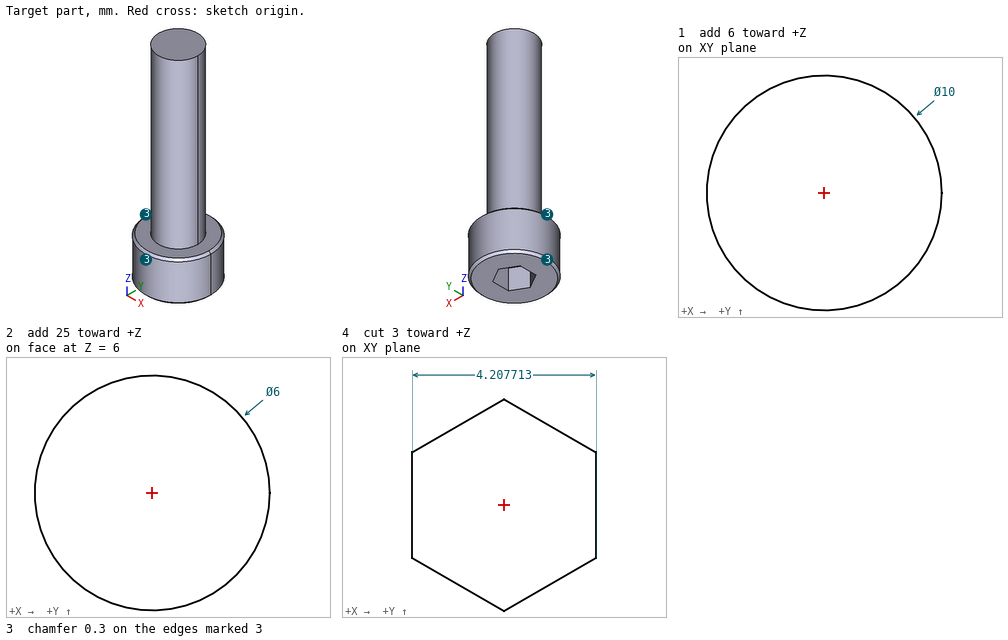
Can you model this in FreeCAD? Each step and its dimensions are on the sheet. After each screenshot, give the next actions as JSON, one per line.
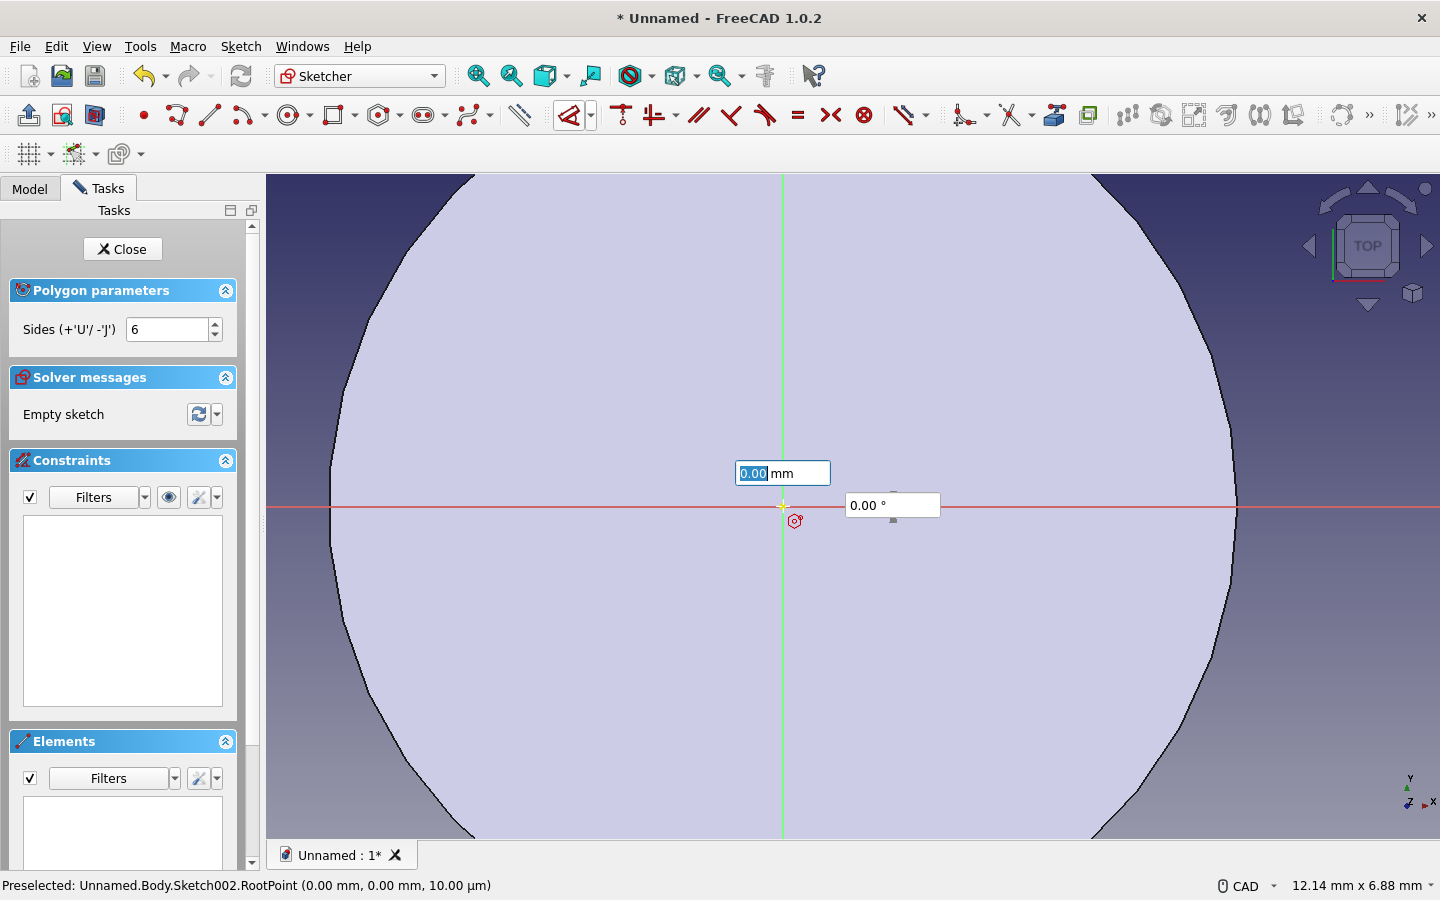
{"action": "left_click", "coordinate": [783, 272]}
{"action": "right_click", "coordinate": [783, 272]}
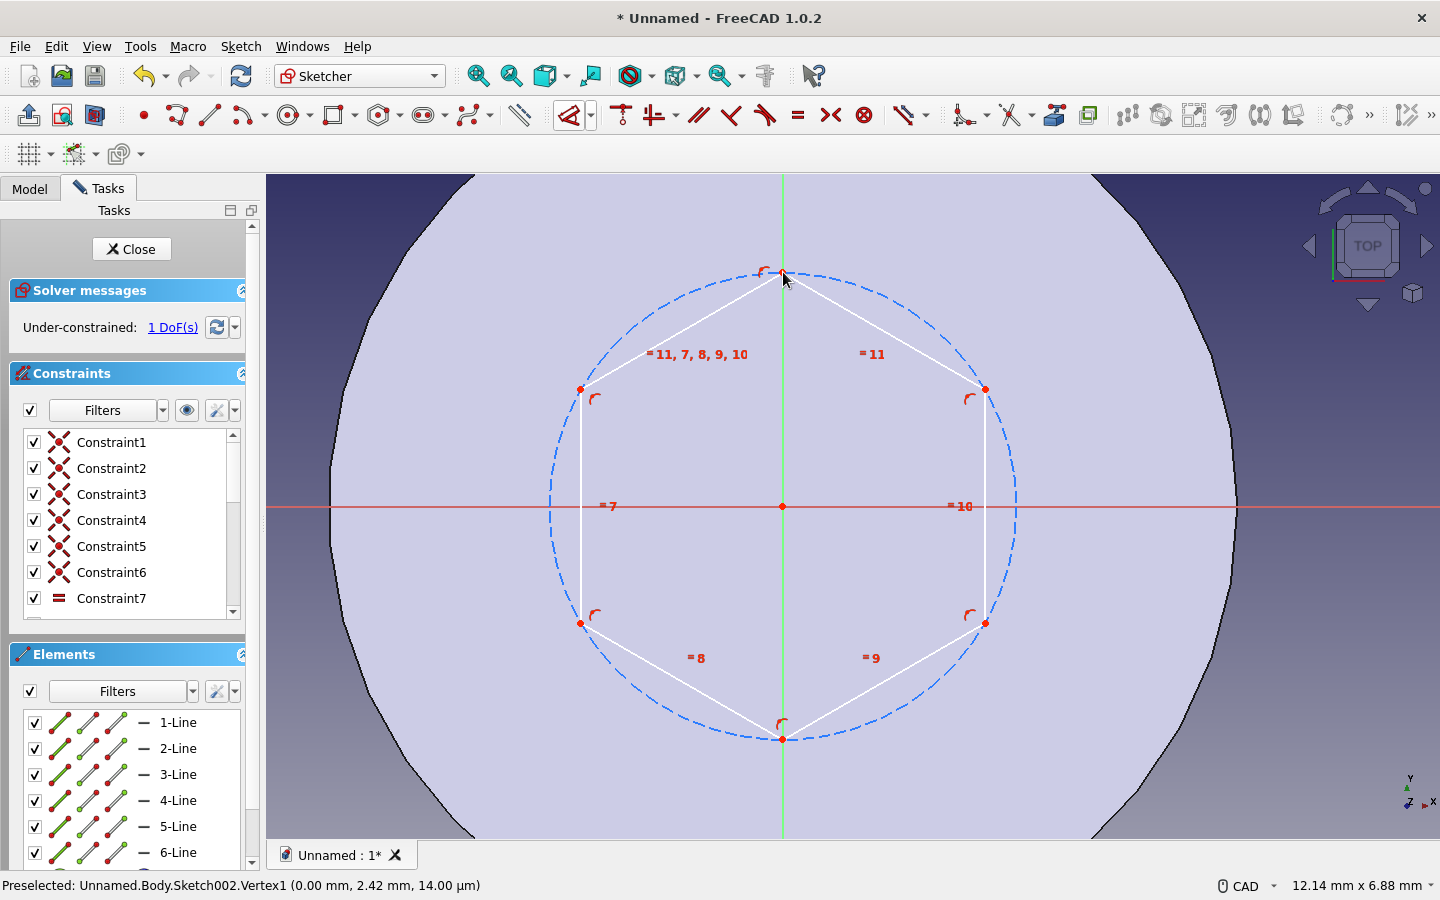
{"action": "key", "text": "d"}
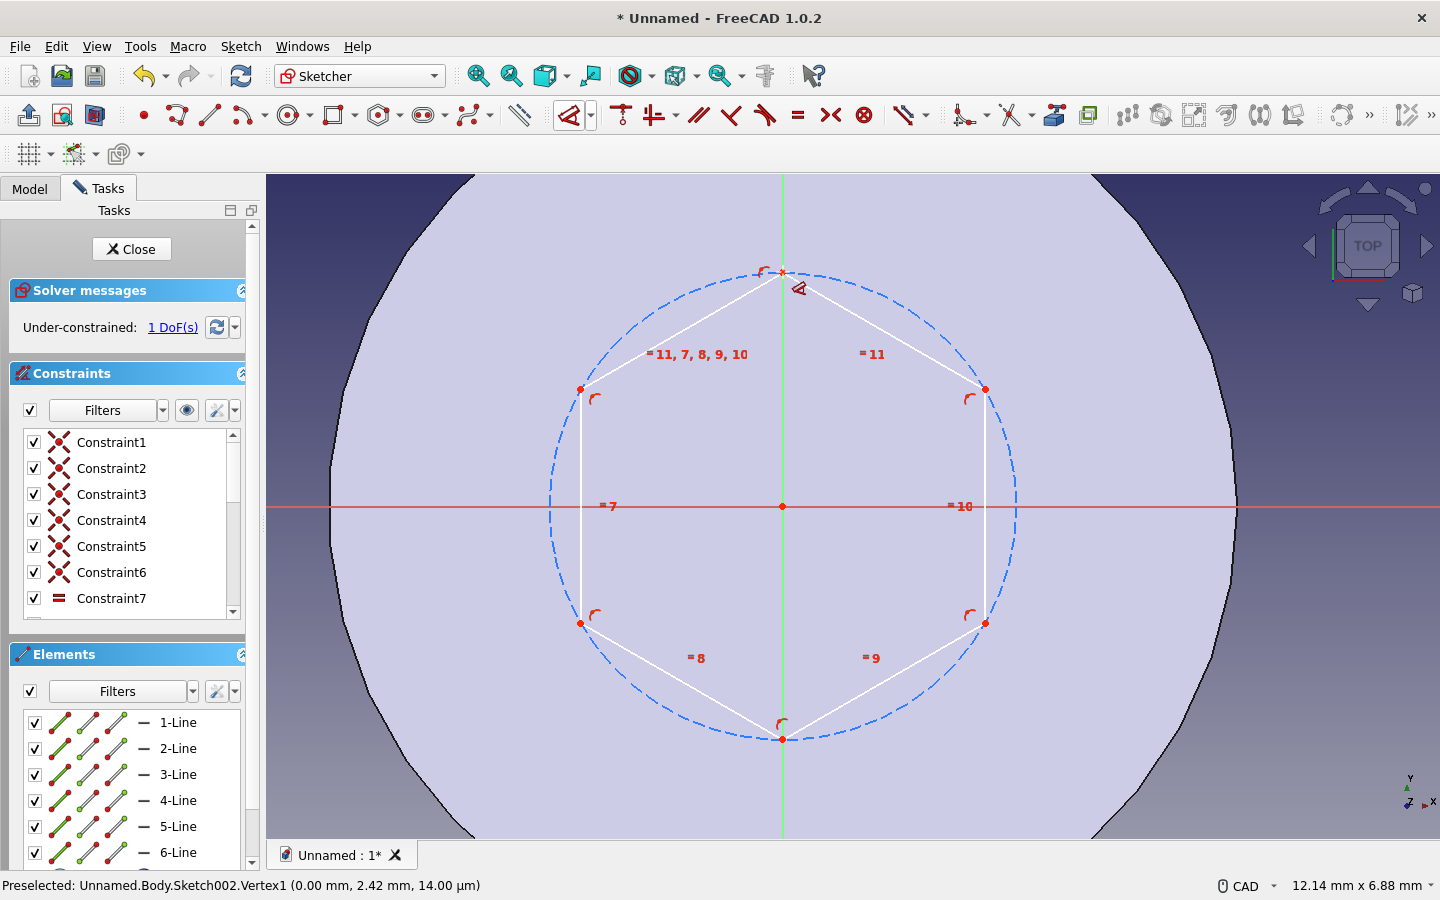
{"action": "left_click", "coordinate": [581, 390]}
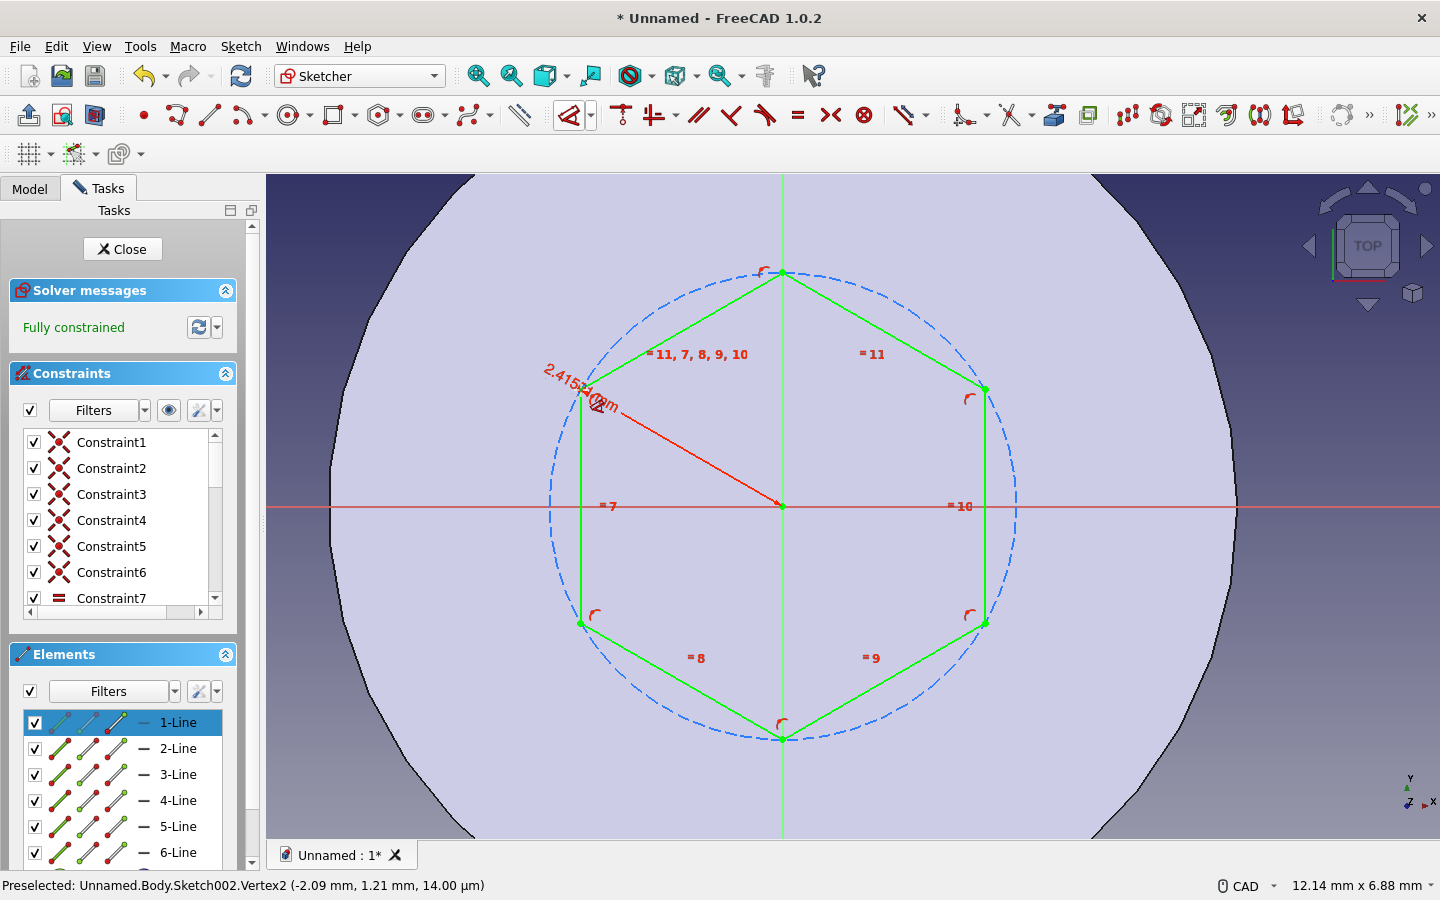
{"action": "left_click", "coordinate": [985, 623]}
{"action": "left_click", "coordinate": [690, 657]}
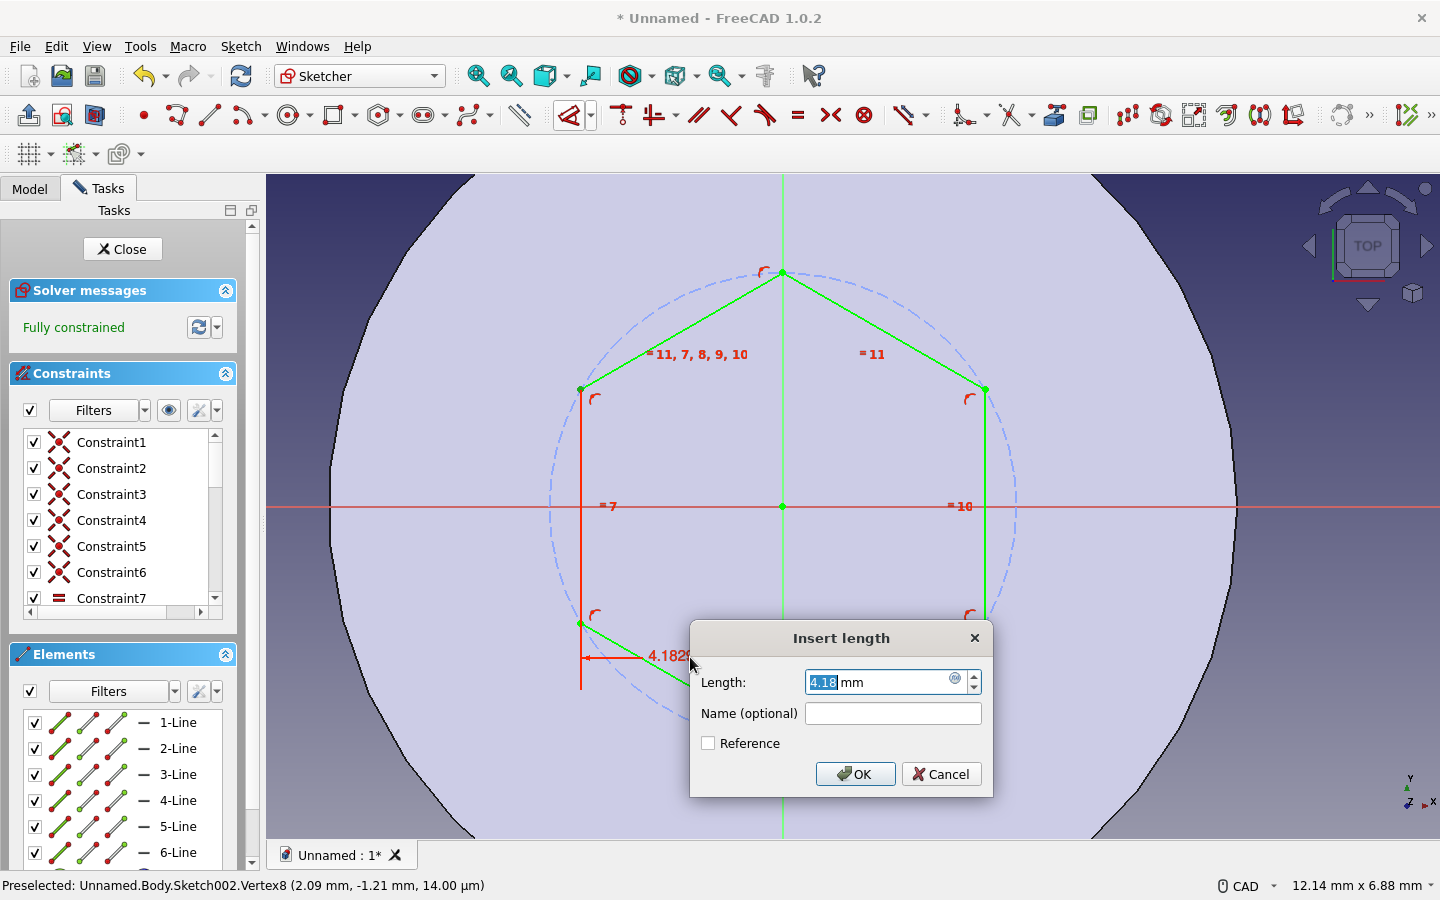
{"action": "type", "text": "4.207713"}
{"action": "key", "text": "Return"}
{"action": "key", "text": "Escape"}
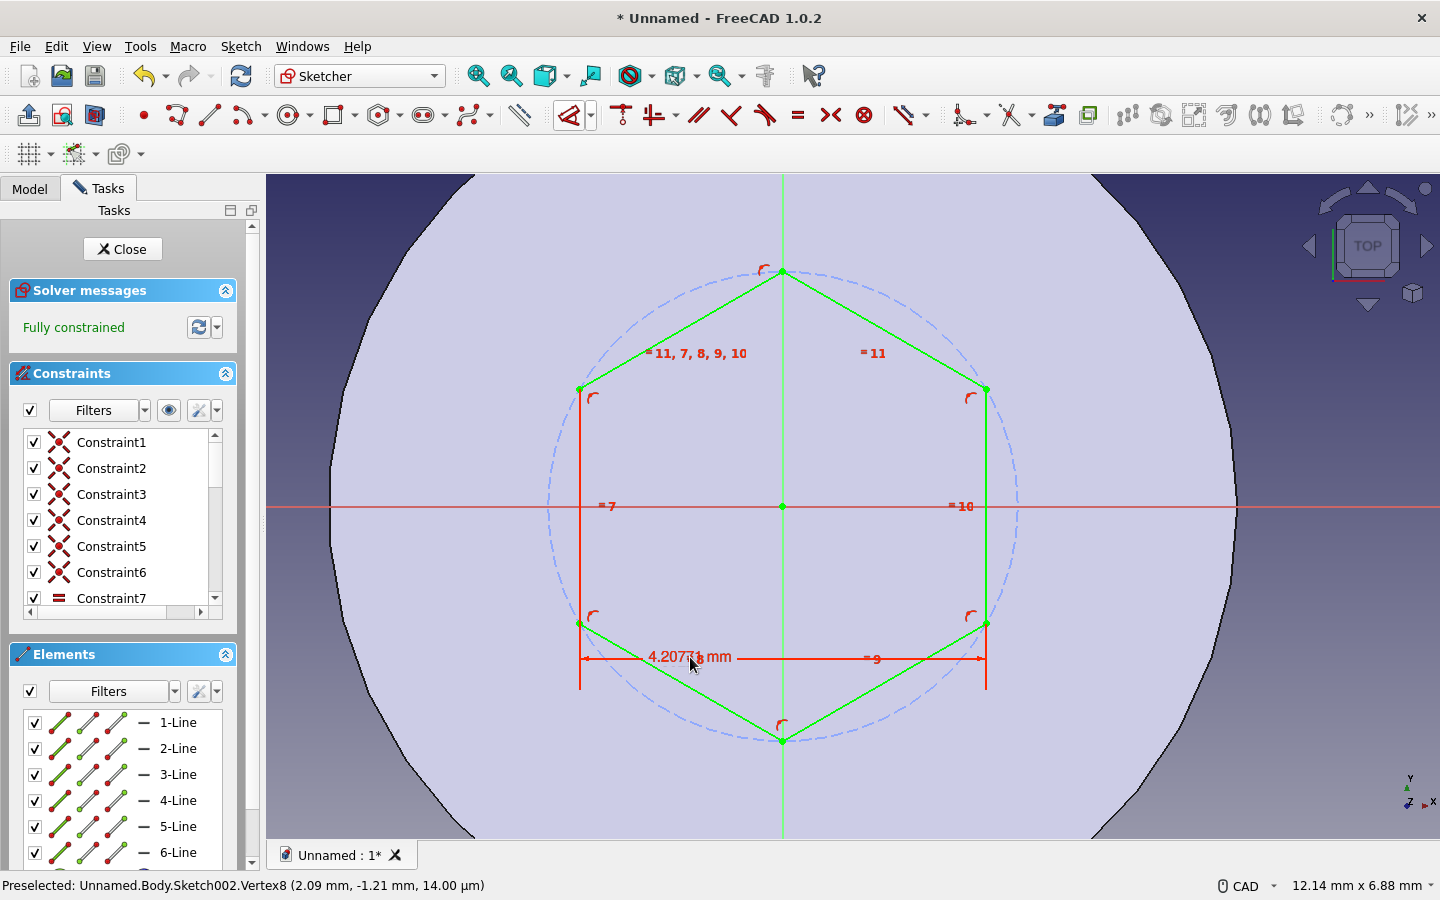
{"action": "left_click", "coordinate": [123, 249]}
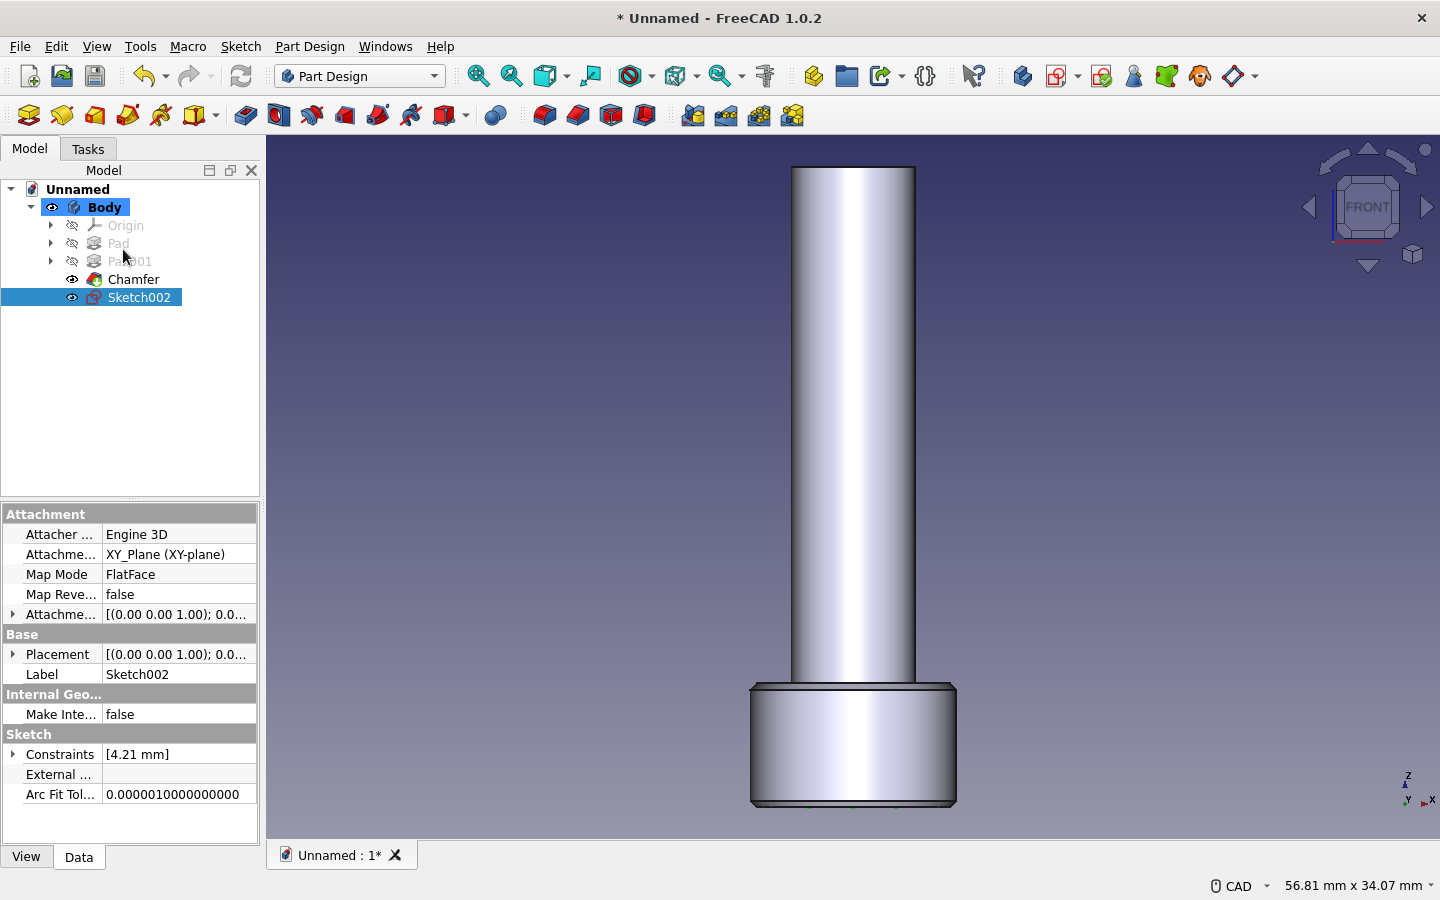
{"action": "left_click", "coordinate": [246, 116]}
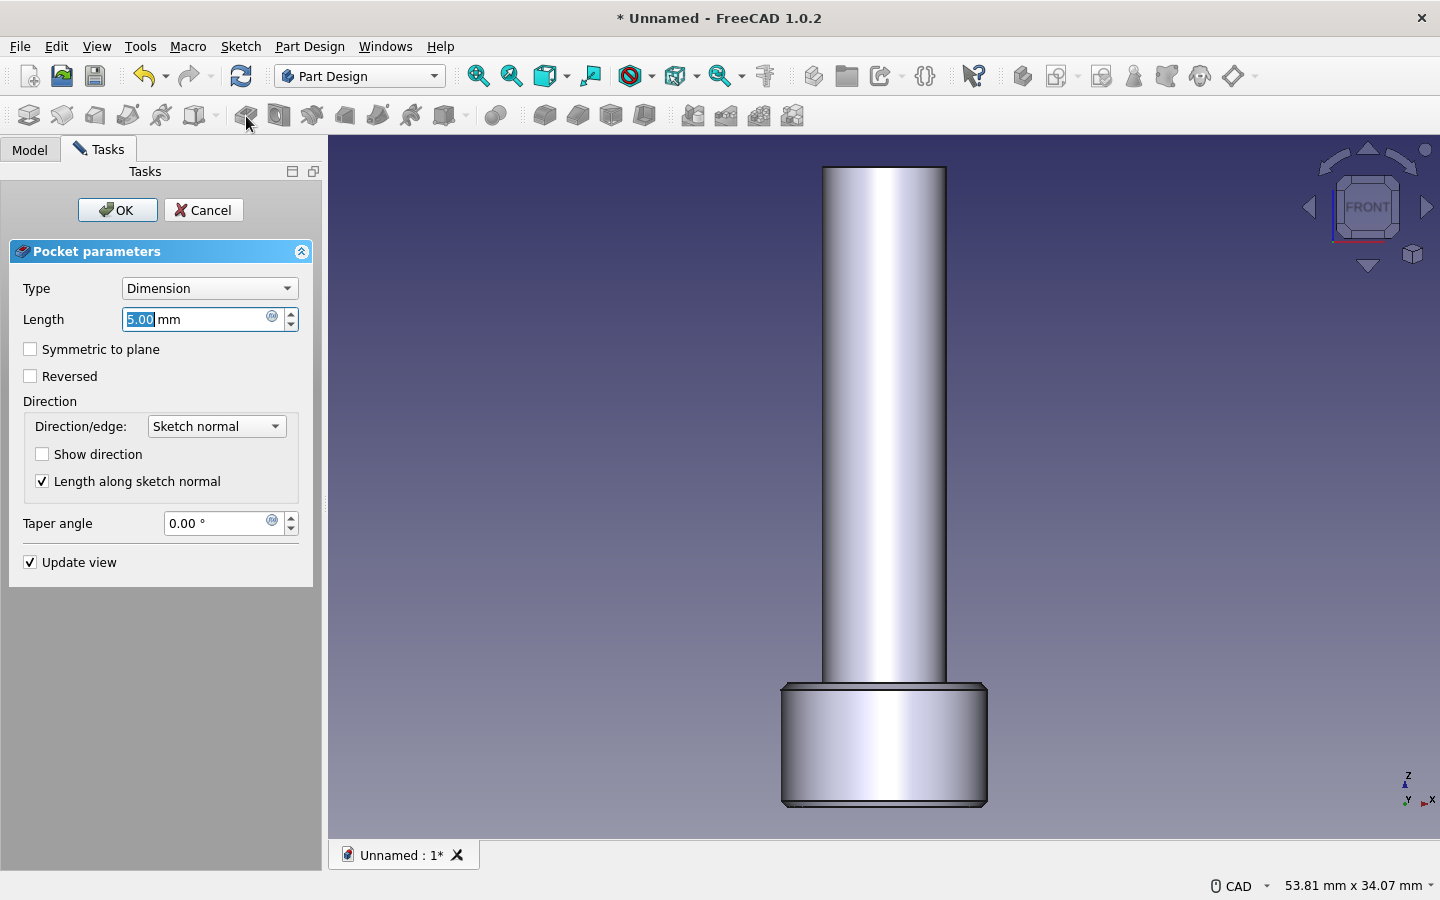
{"action": "type", "text": "3"}
{"action": "key", "text": "Tab"}